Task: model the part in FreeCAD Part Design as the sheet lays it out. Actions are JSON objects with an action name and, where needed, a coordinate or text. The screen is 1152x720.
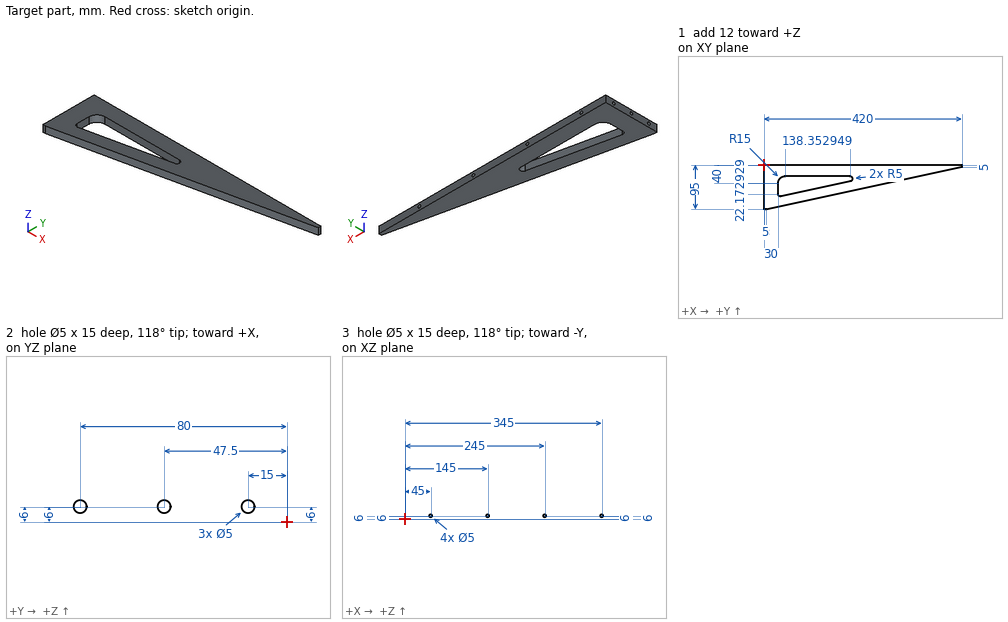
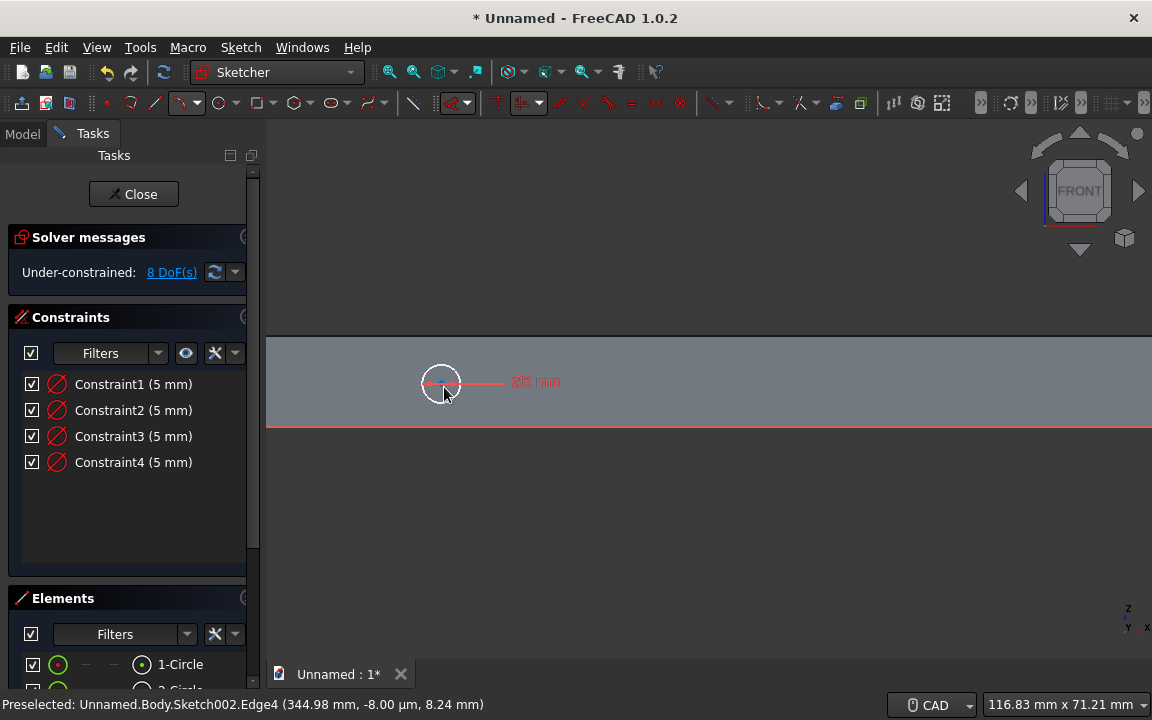
{"action": "left_click", "coordinate": [441, 384]}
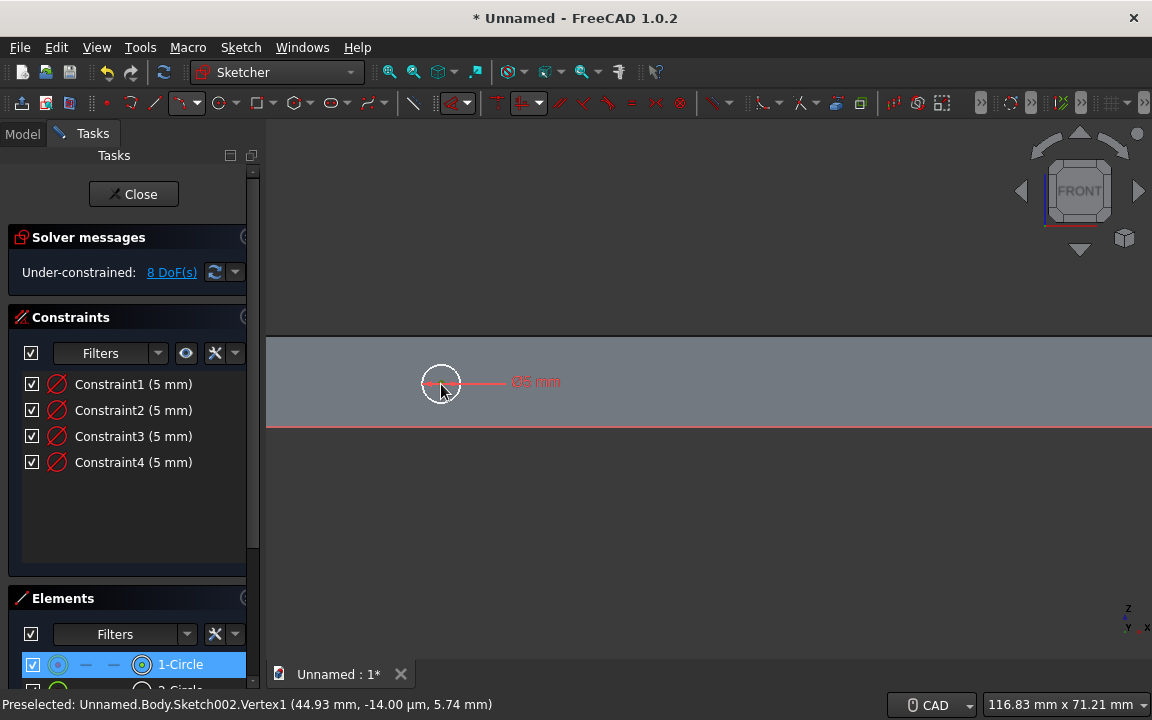
{"action": "left_click", "coordinate": [470, 104]}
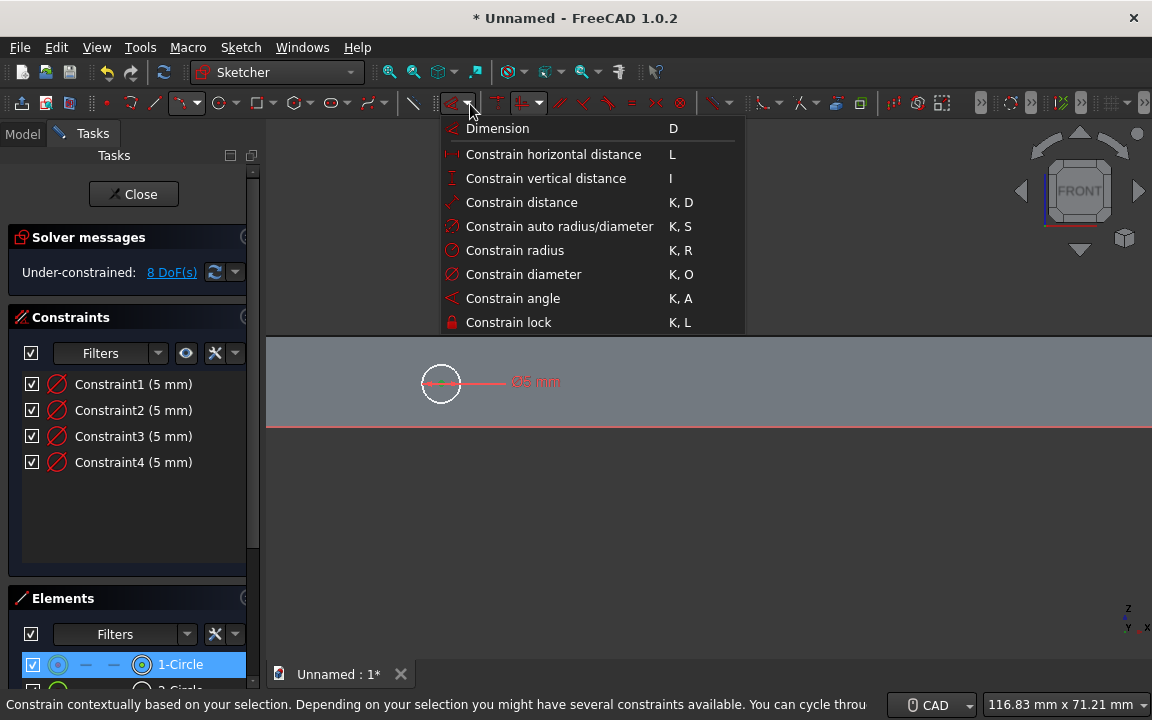
{"action": "left_click", "coordinate": [593, 178]}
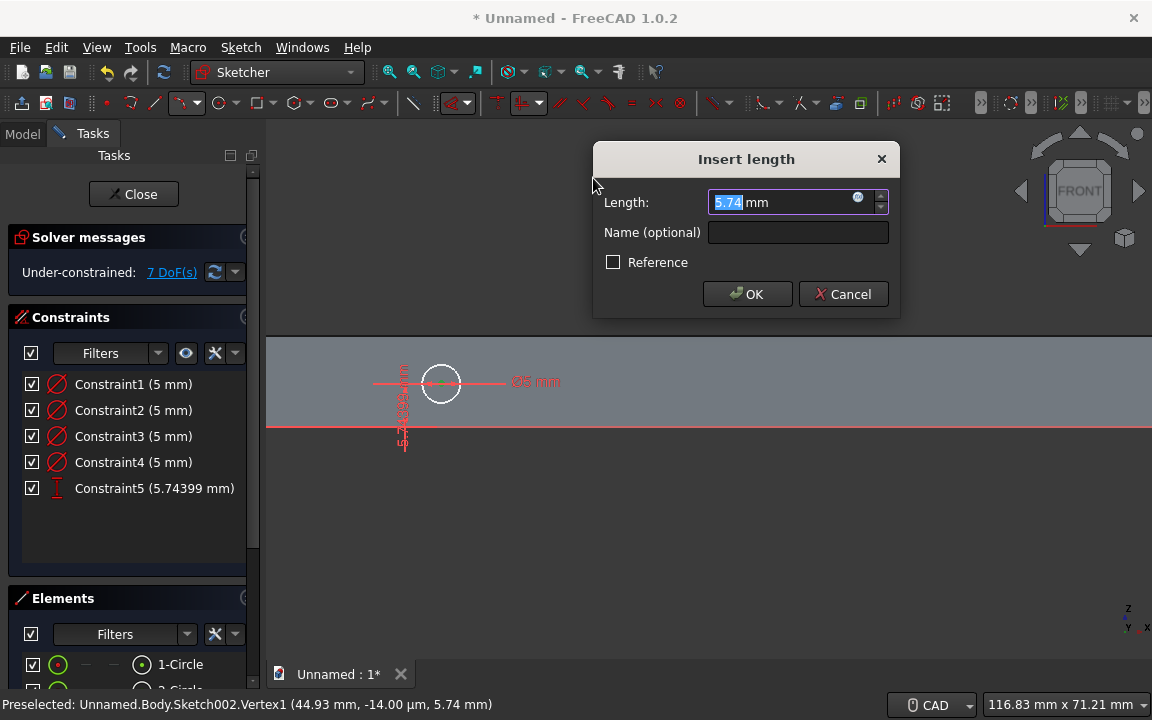
{"action": "type", "text": "6"}
{"action": "key", "text": "Return"}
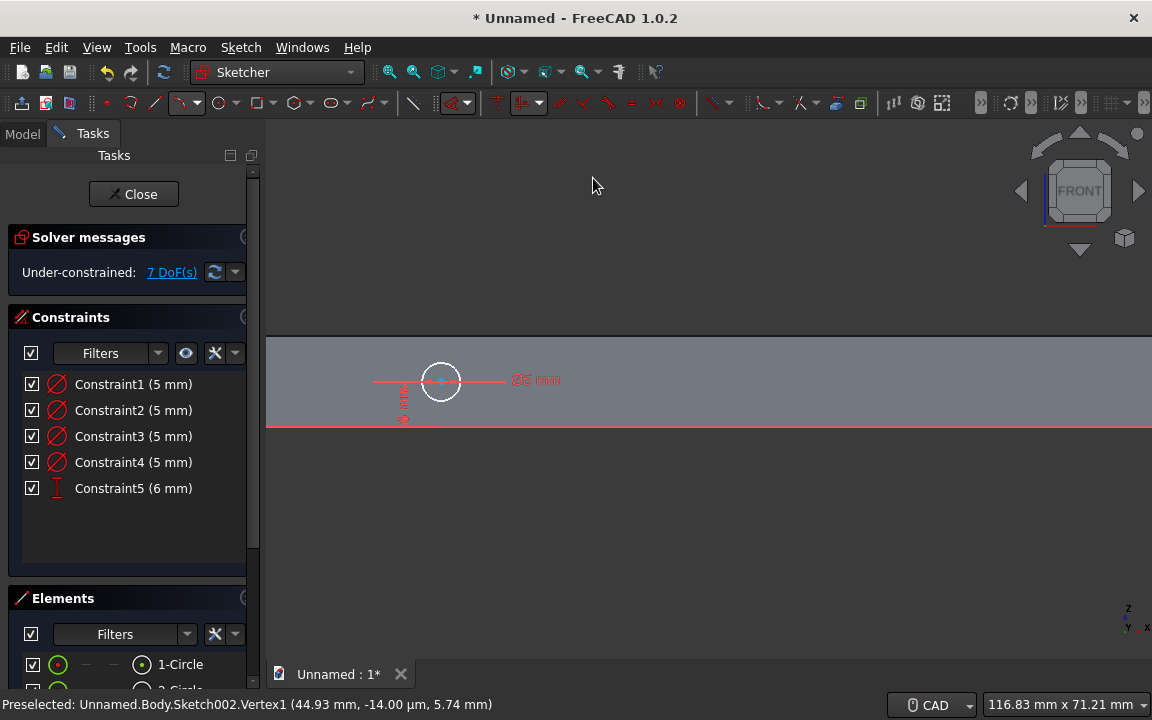
{"action": "scroll", "coordinate": [444, 387], "scroll_direction": "down", "scroll_amount": 8}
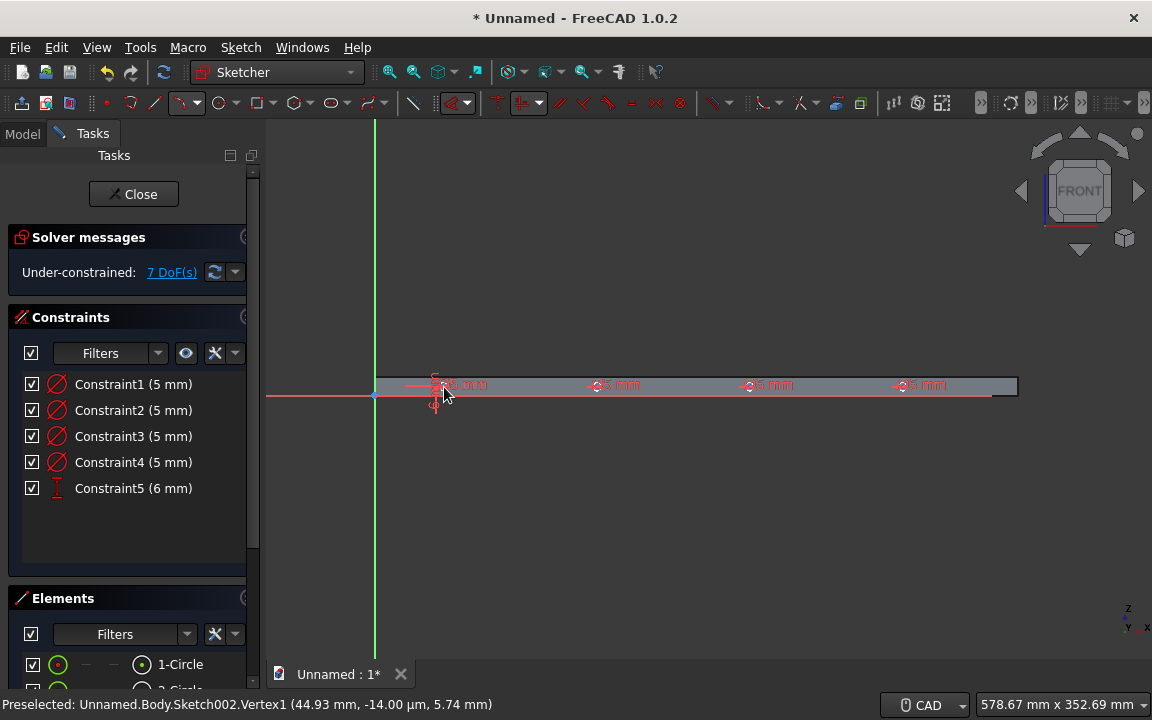
{"action": "scroll", "coordinate": [597, 387], "scroll_direction": "up", "scroll_amount": 8}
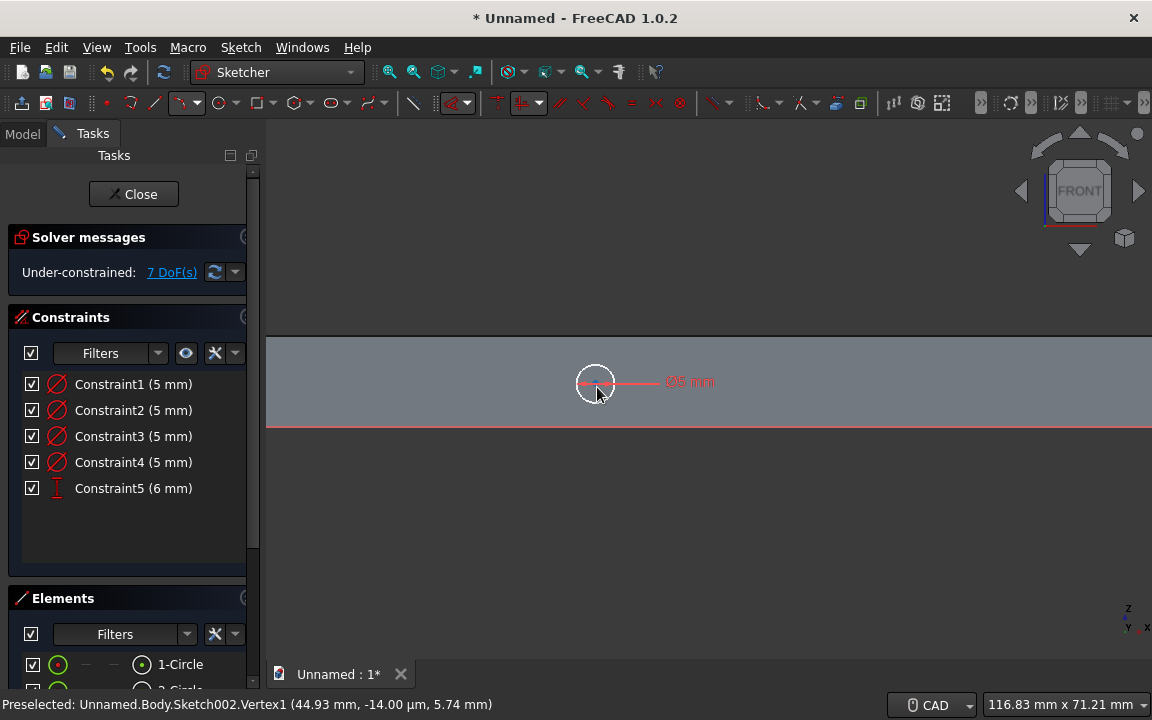
{"action": "left_click", "coordinate": [596, 384]}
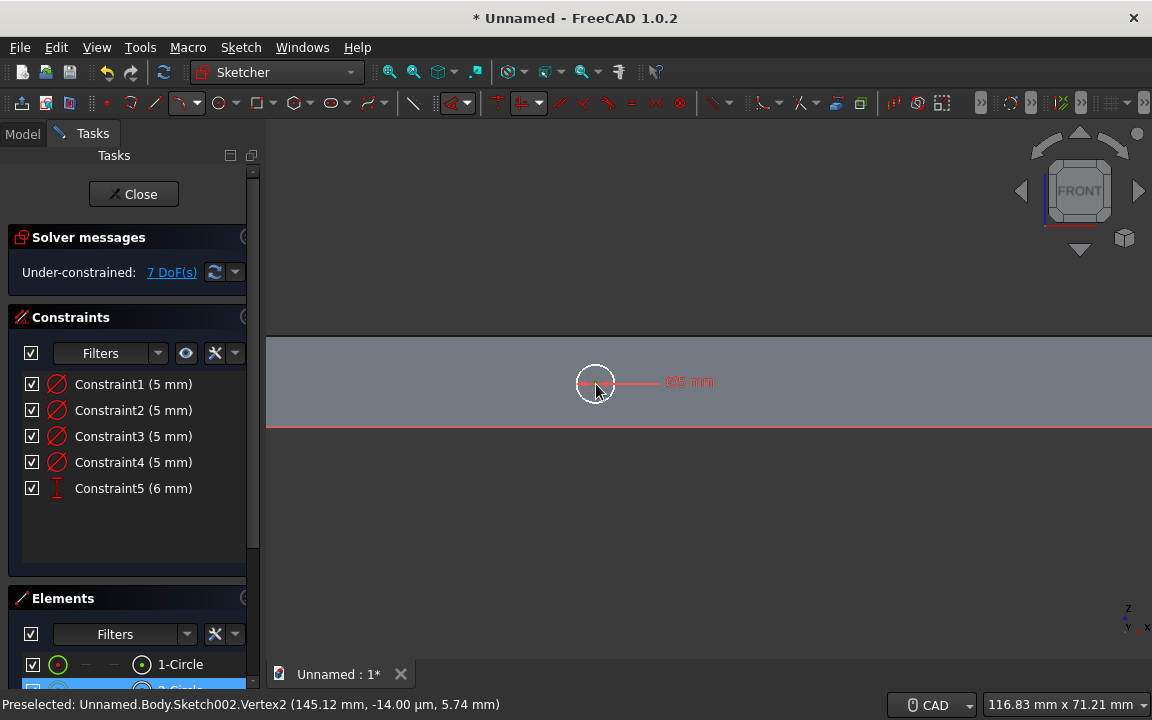
{"action": "left_click", "coordinate": [470, 104]}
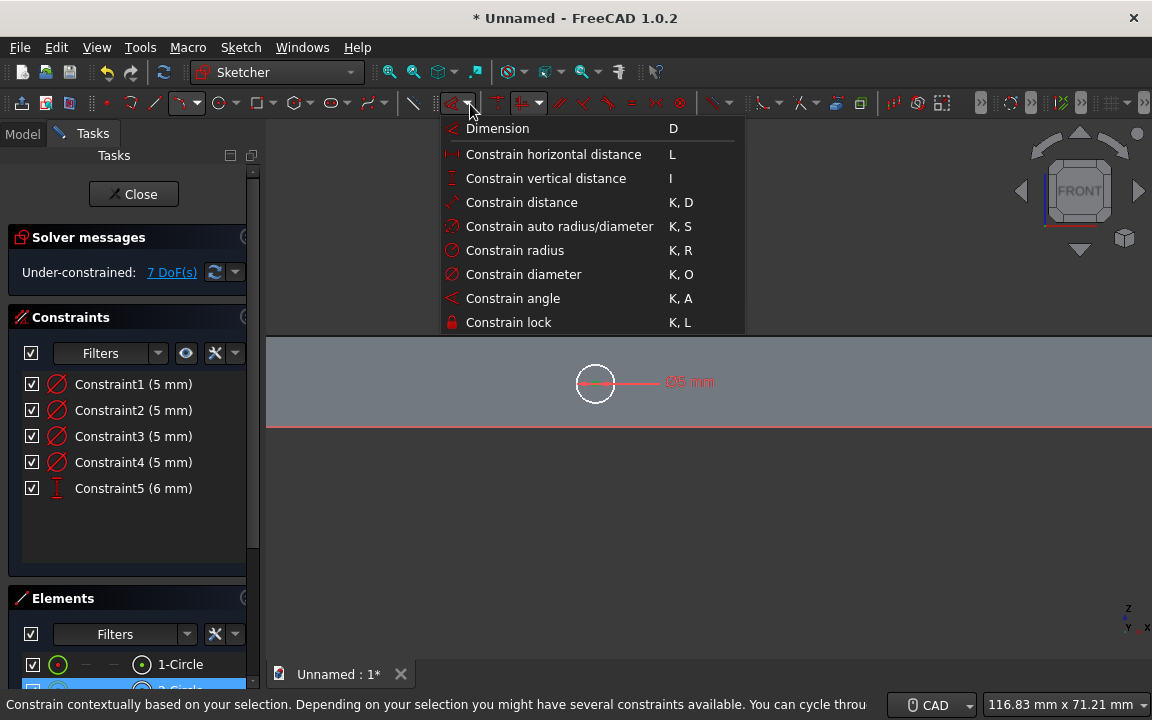
{"action": "left_click", "coordinate": [593, 178]}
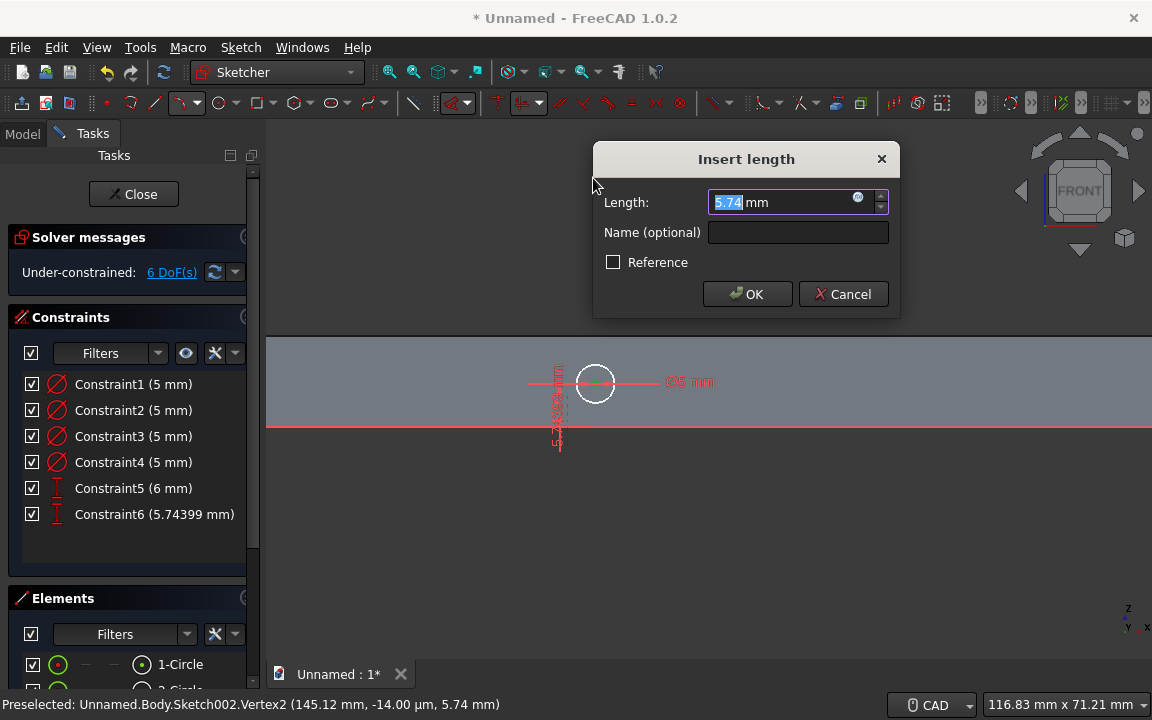
{"action": "type", "text": "6"}
{"action": "key", "text": "Return"}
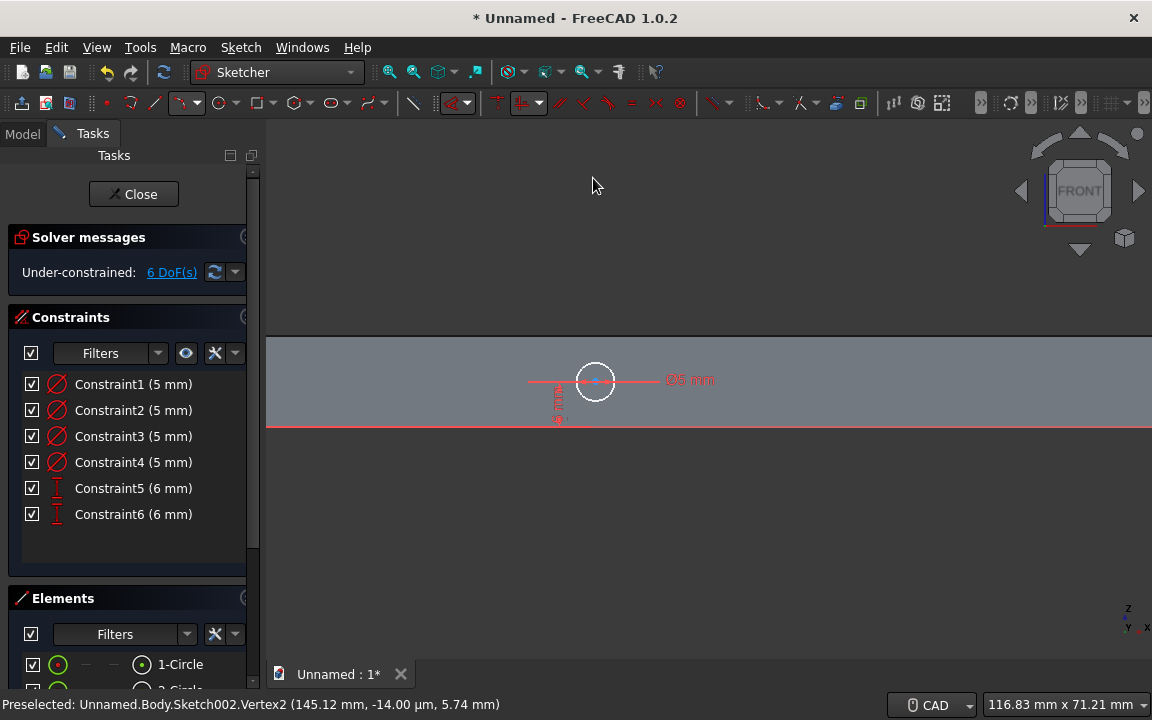
{"action": "scroll", "coordinate": [597, 387], "scroll_direction": "down", "scroll_amount": 8}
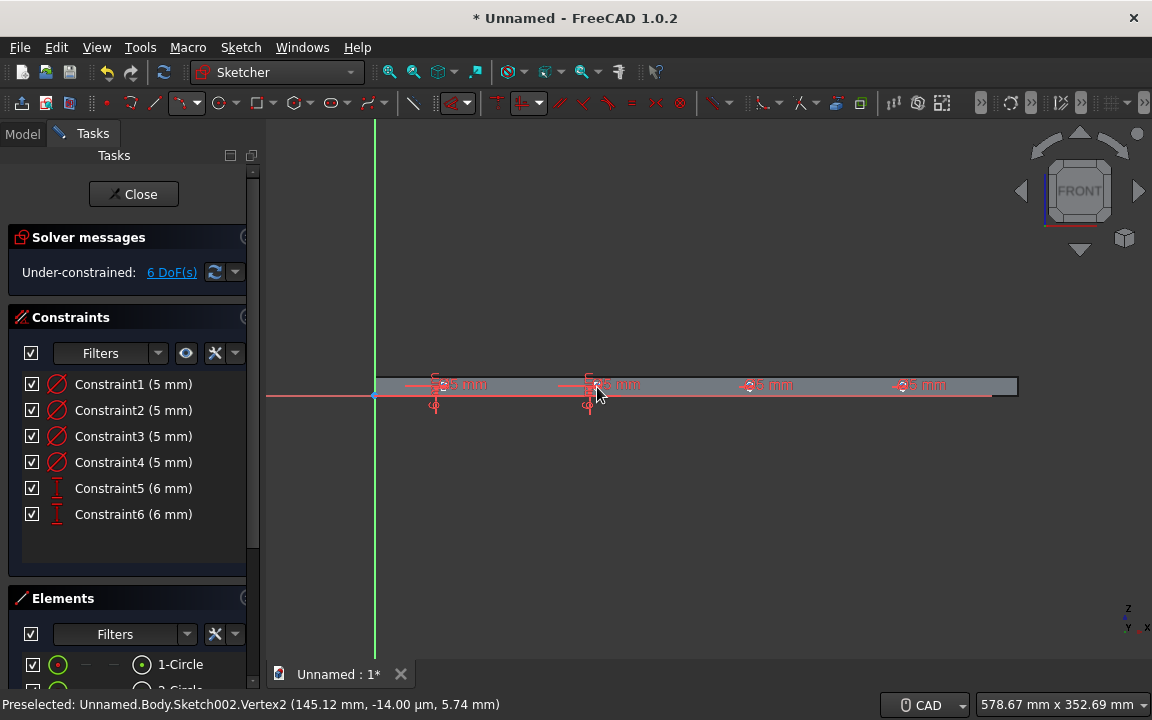
{"action": "scroll", "coordinate": [750, 387], "scroll_direction": "up", "scroll_amount": 8}